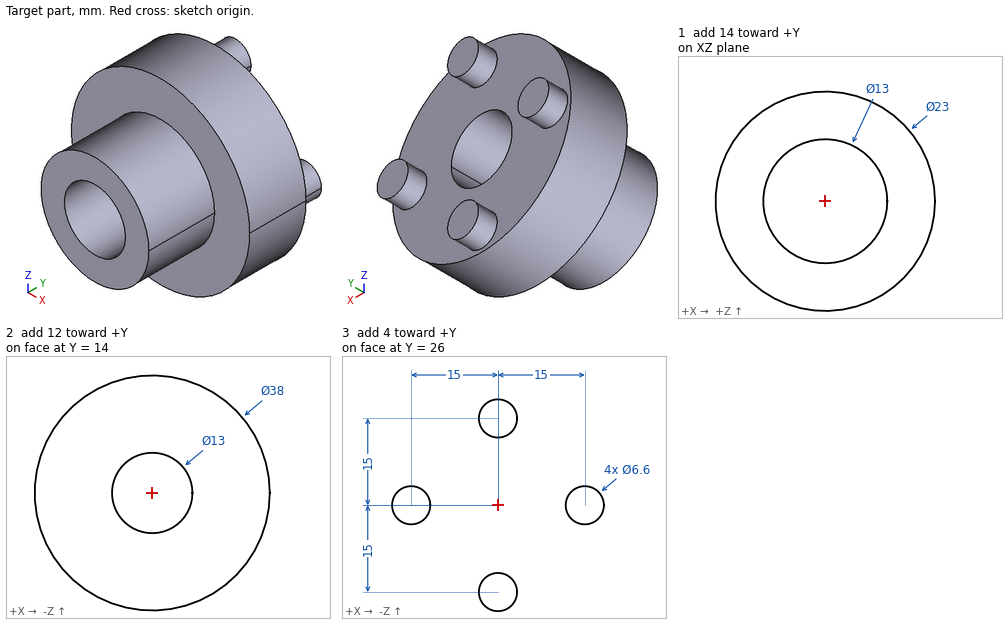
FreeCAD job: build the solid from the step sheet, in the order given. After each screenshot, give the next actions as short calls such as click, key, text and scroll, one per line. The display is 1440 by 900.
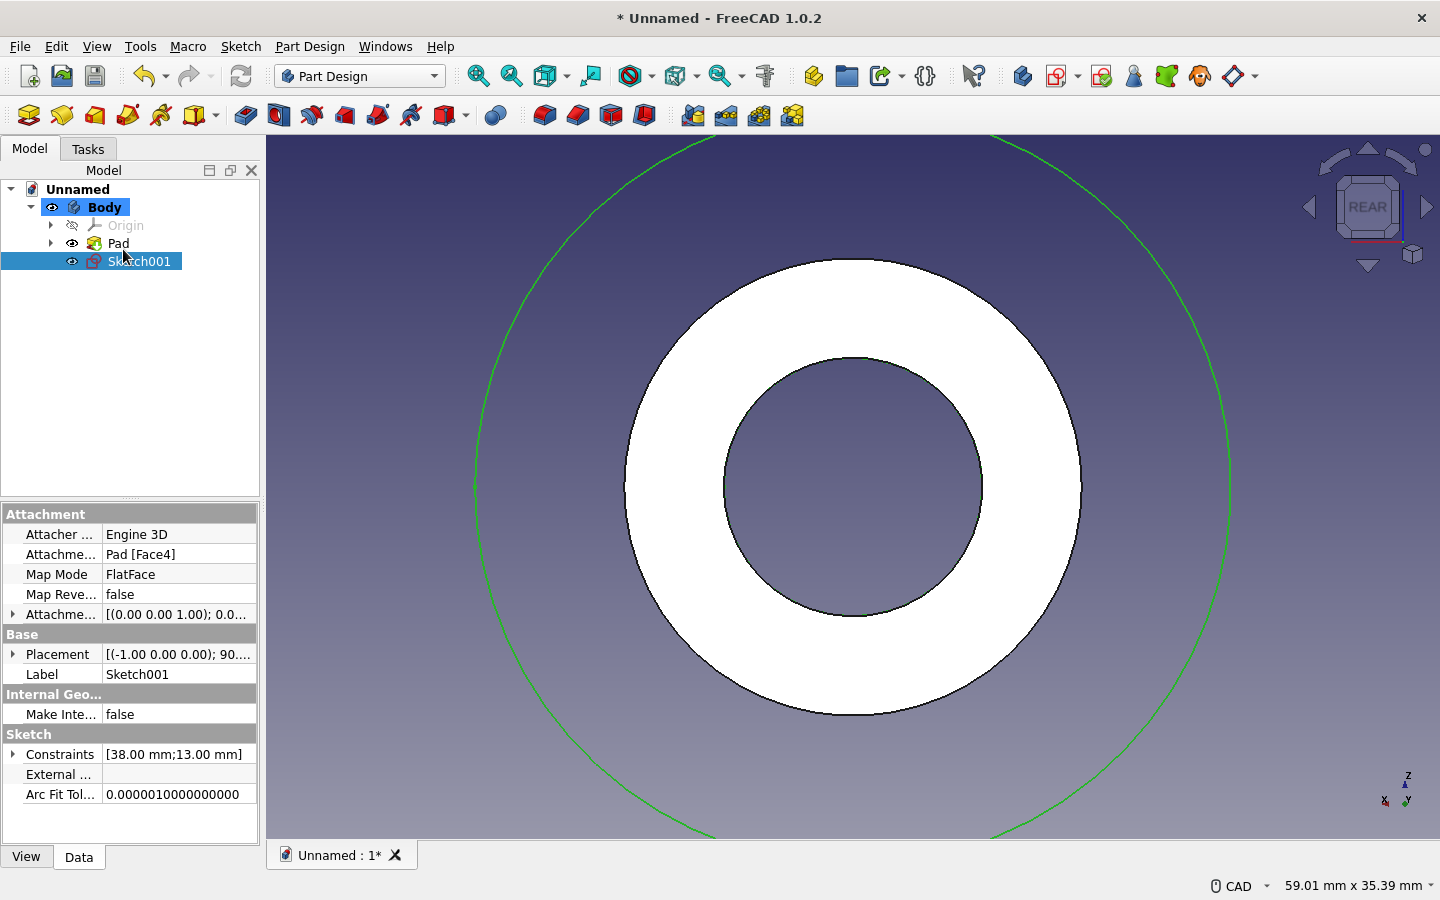
click(29, 116)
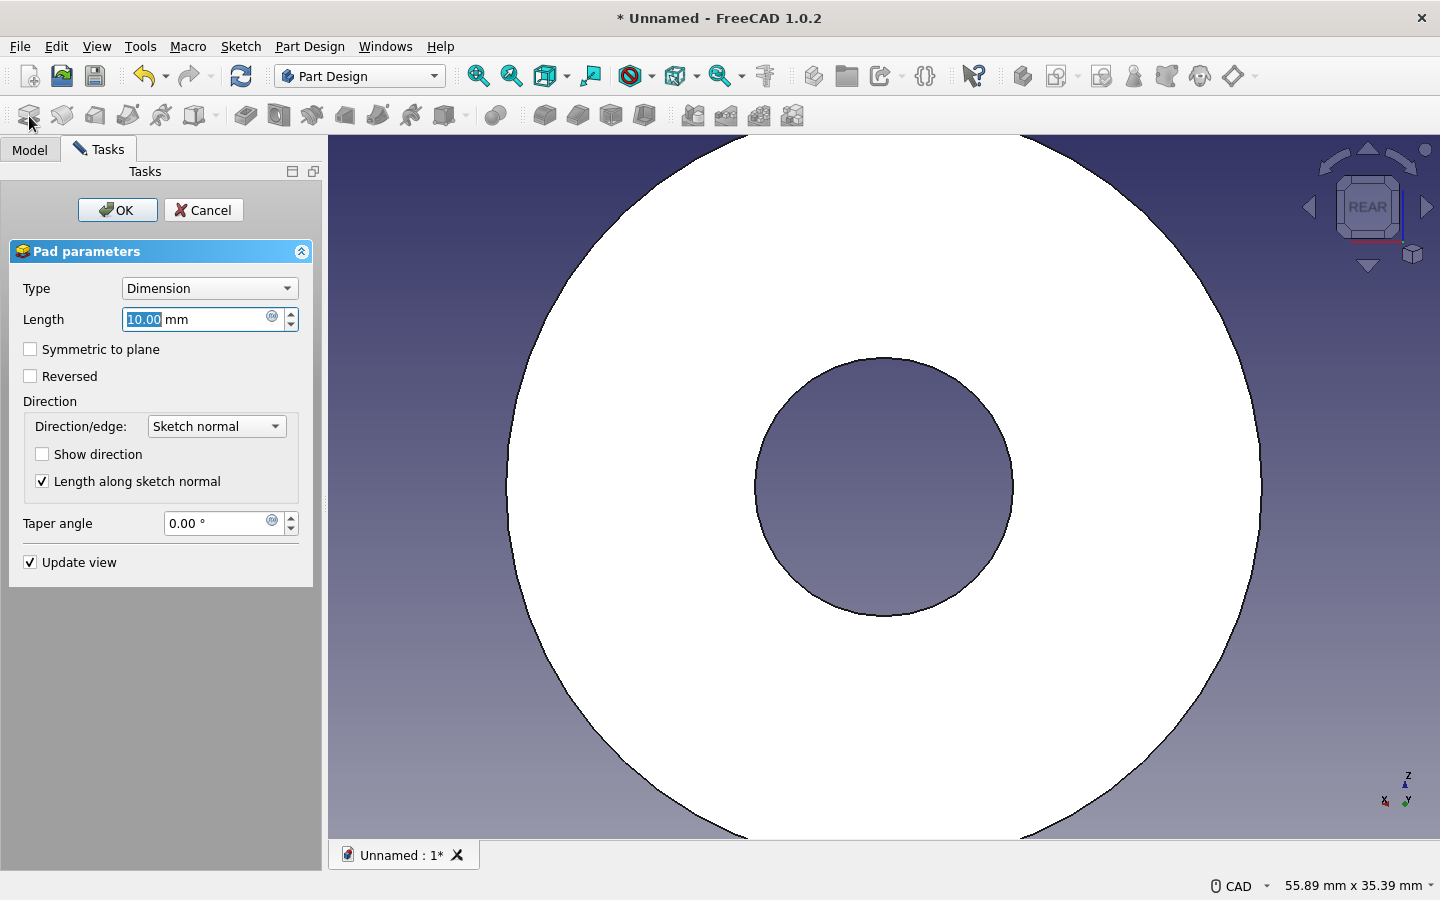
text(12)
key(Tab)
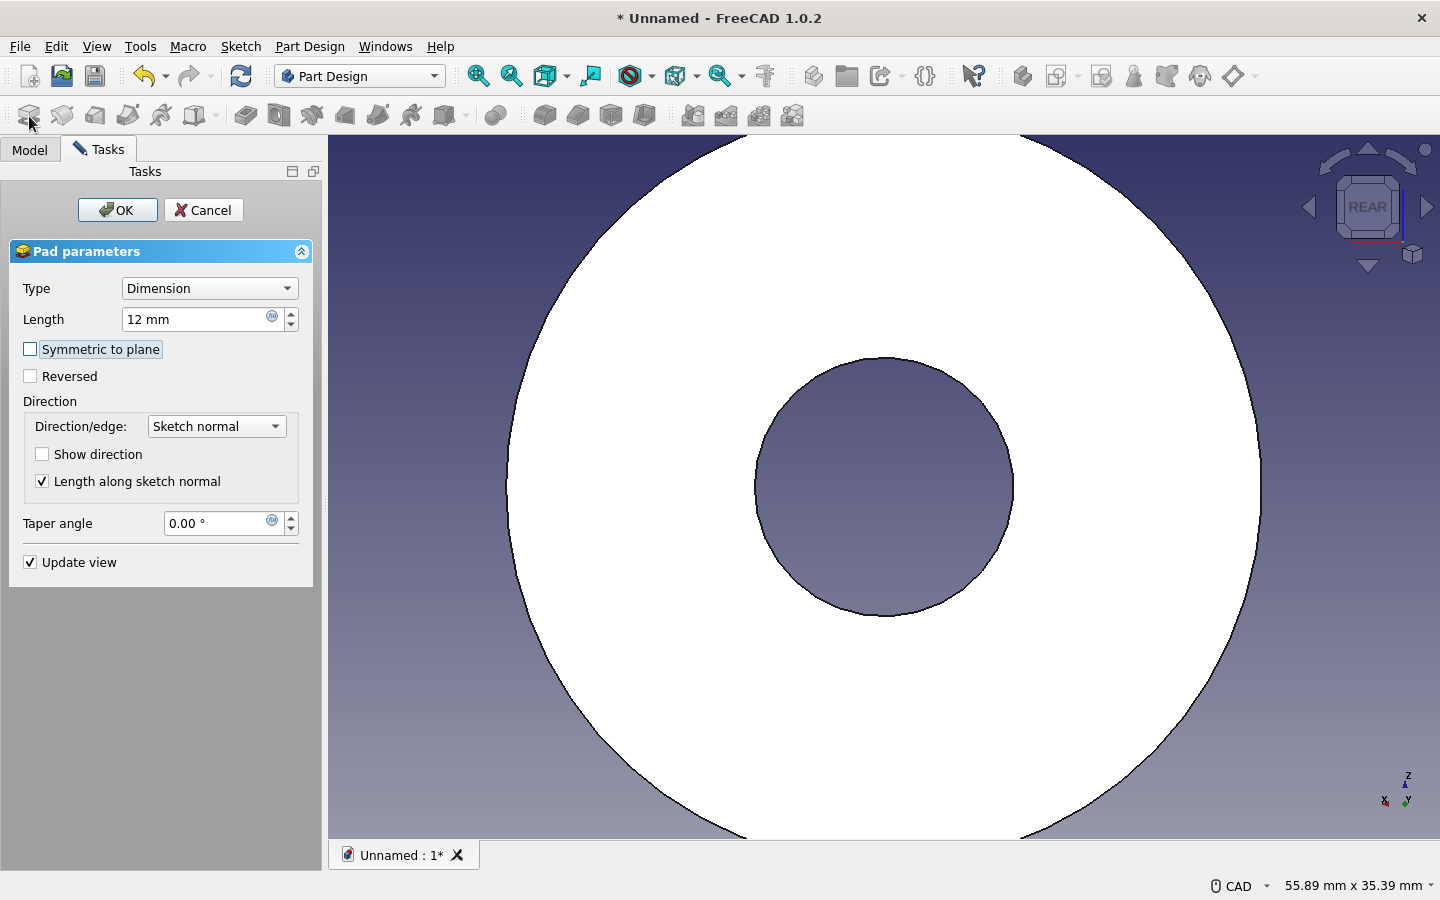
click(118, 210)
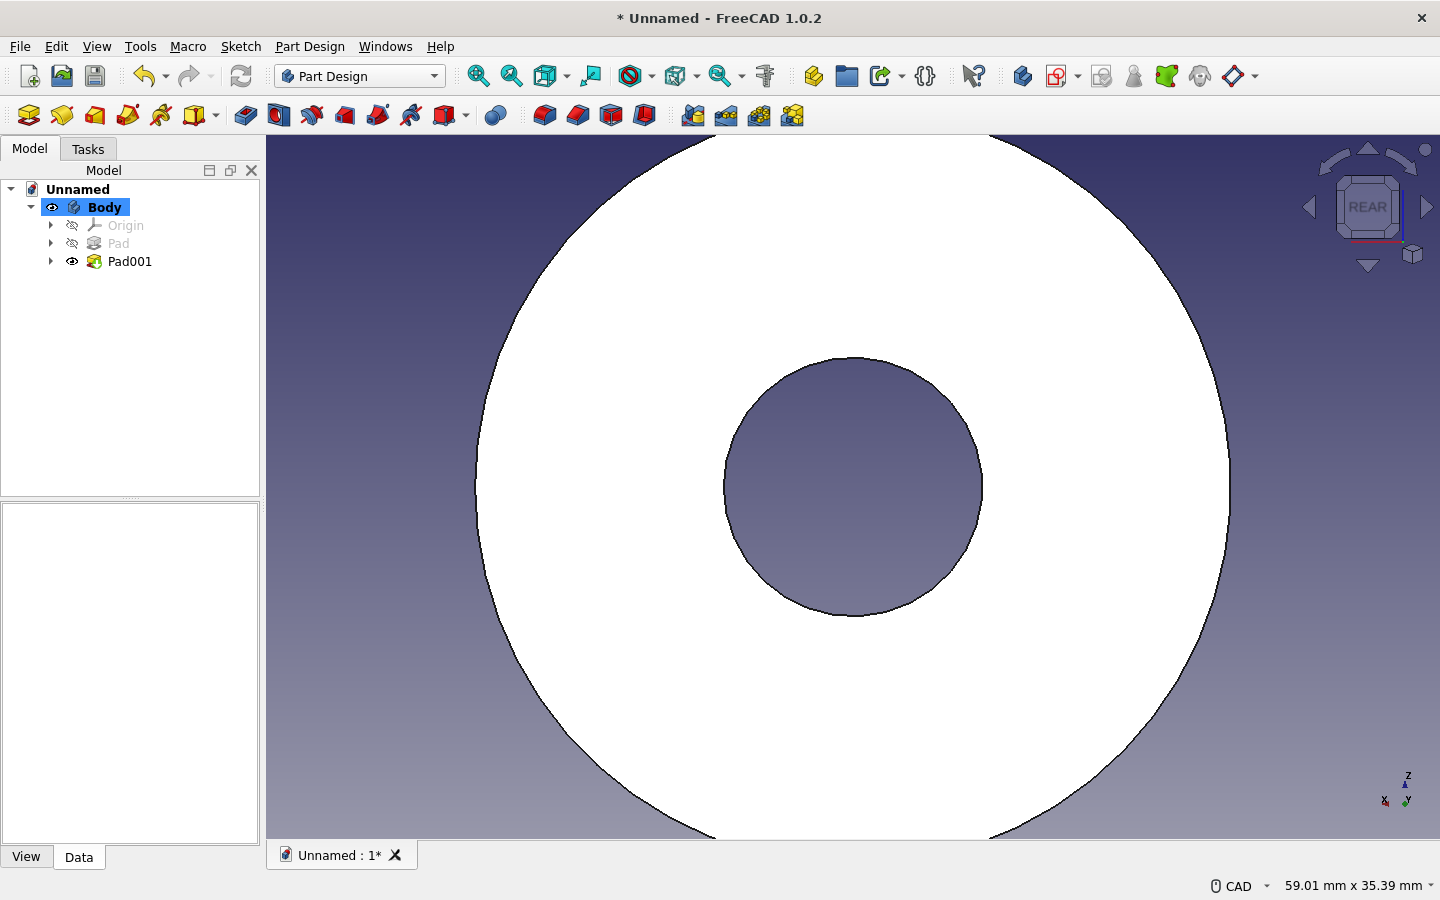
key(v)
key(f)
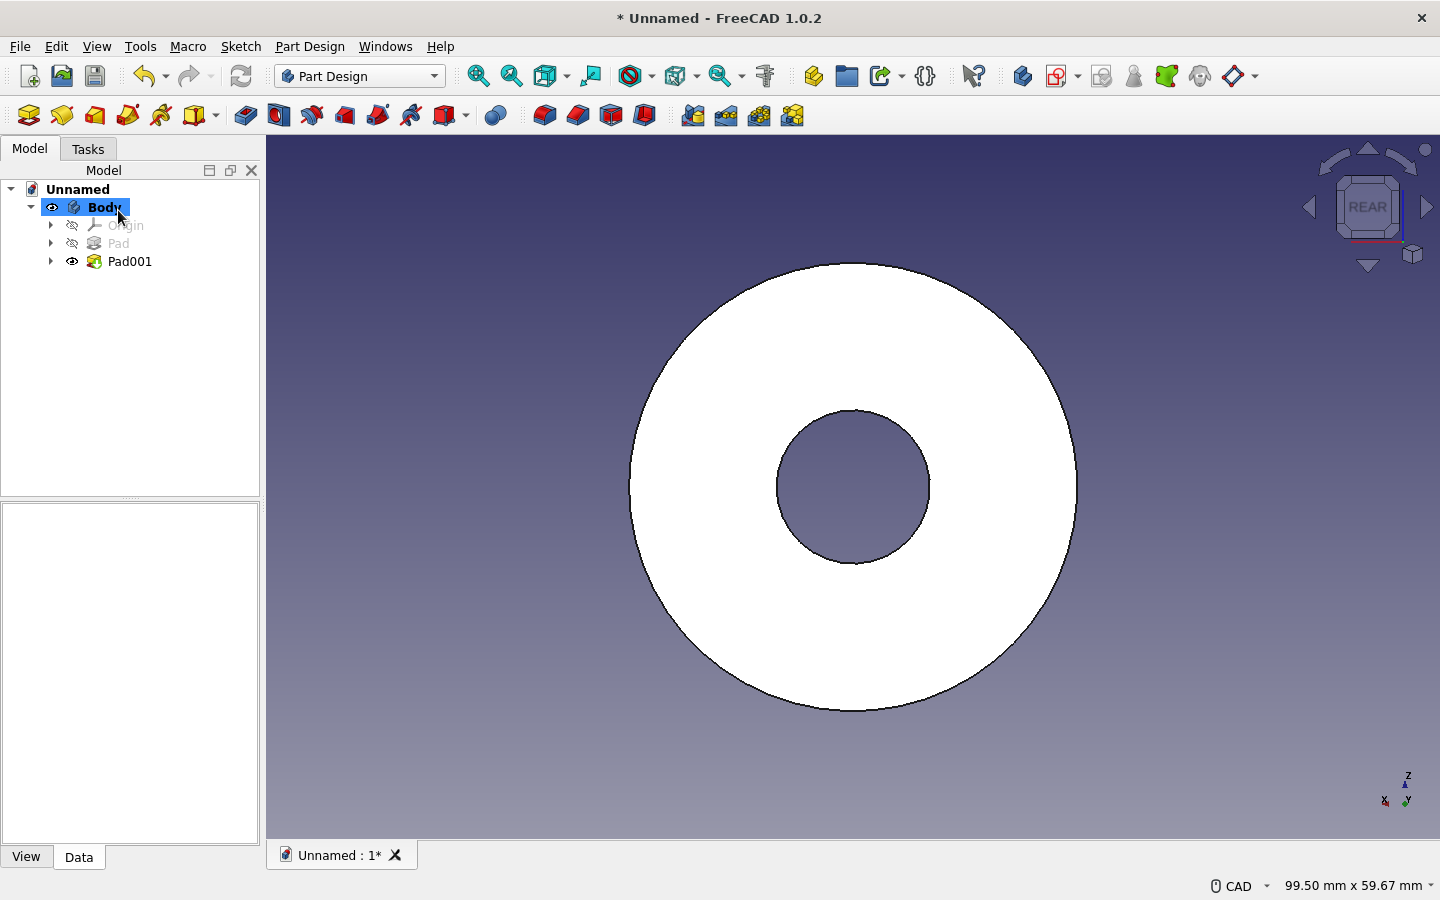
click(917, 614)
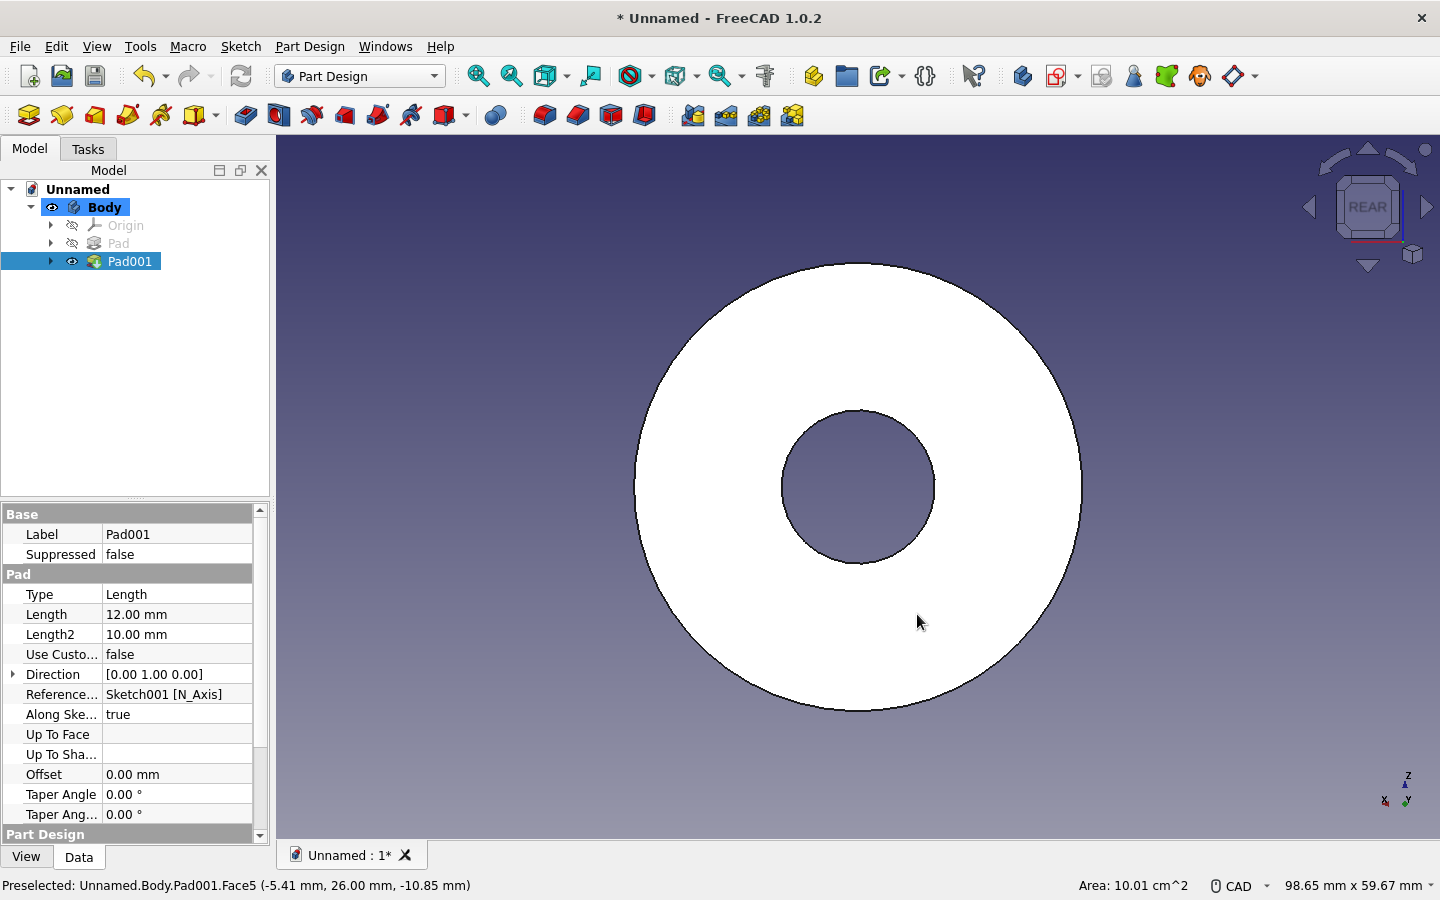
click(1056, 76)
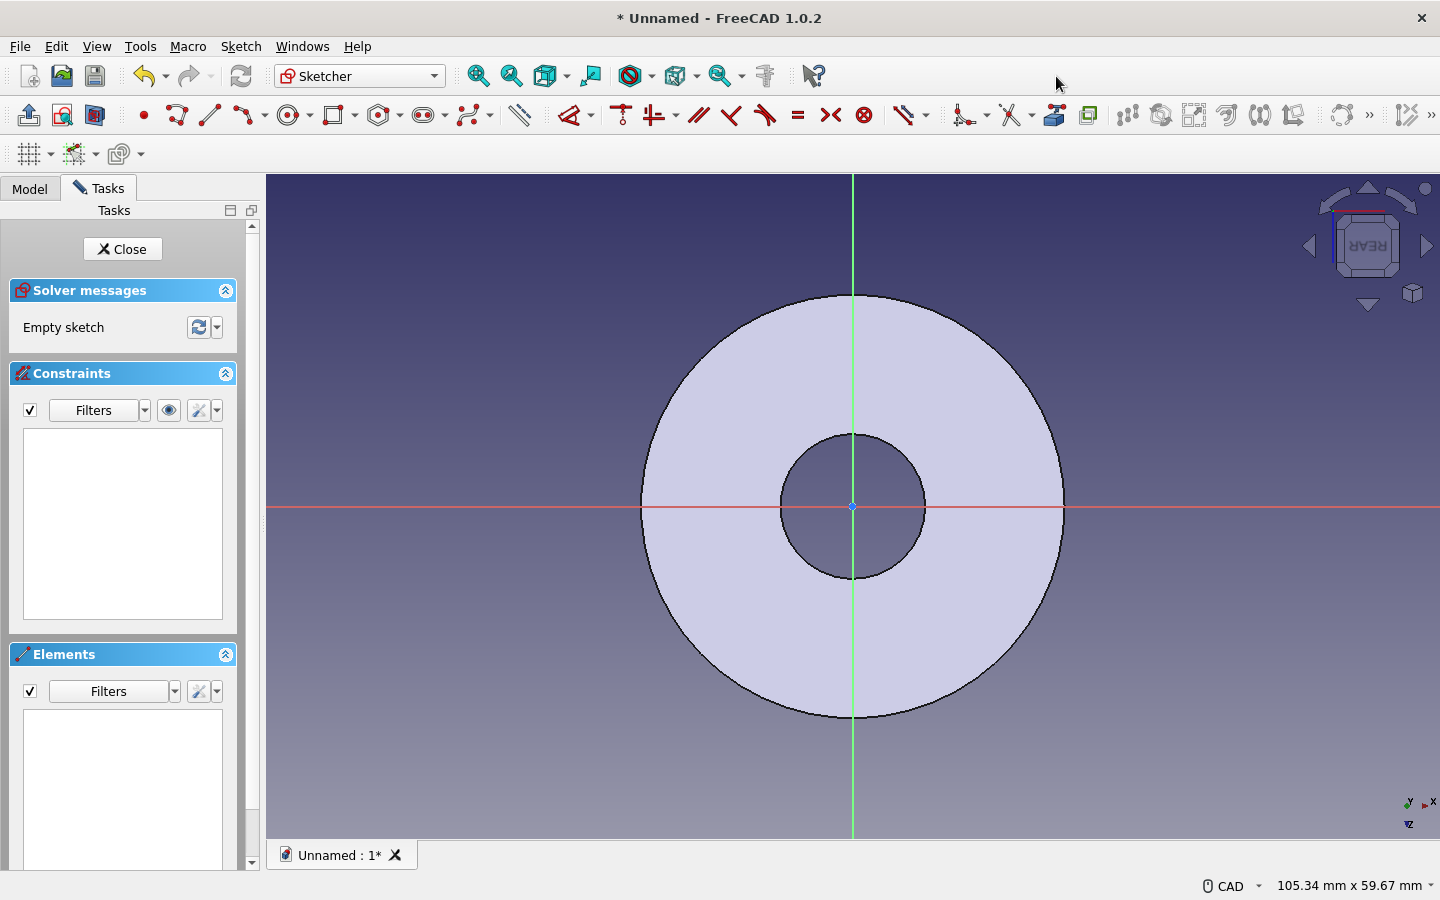
key(g)
key(c)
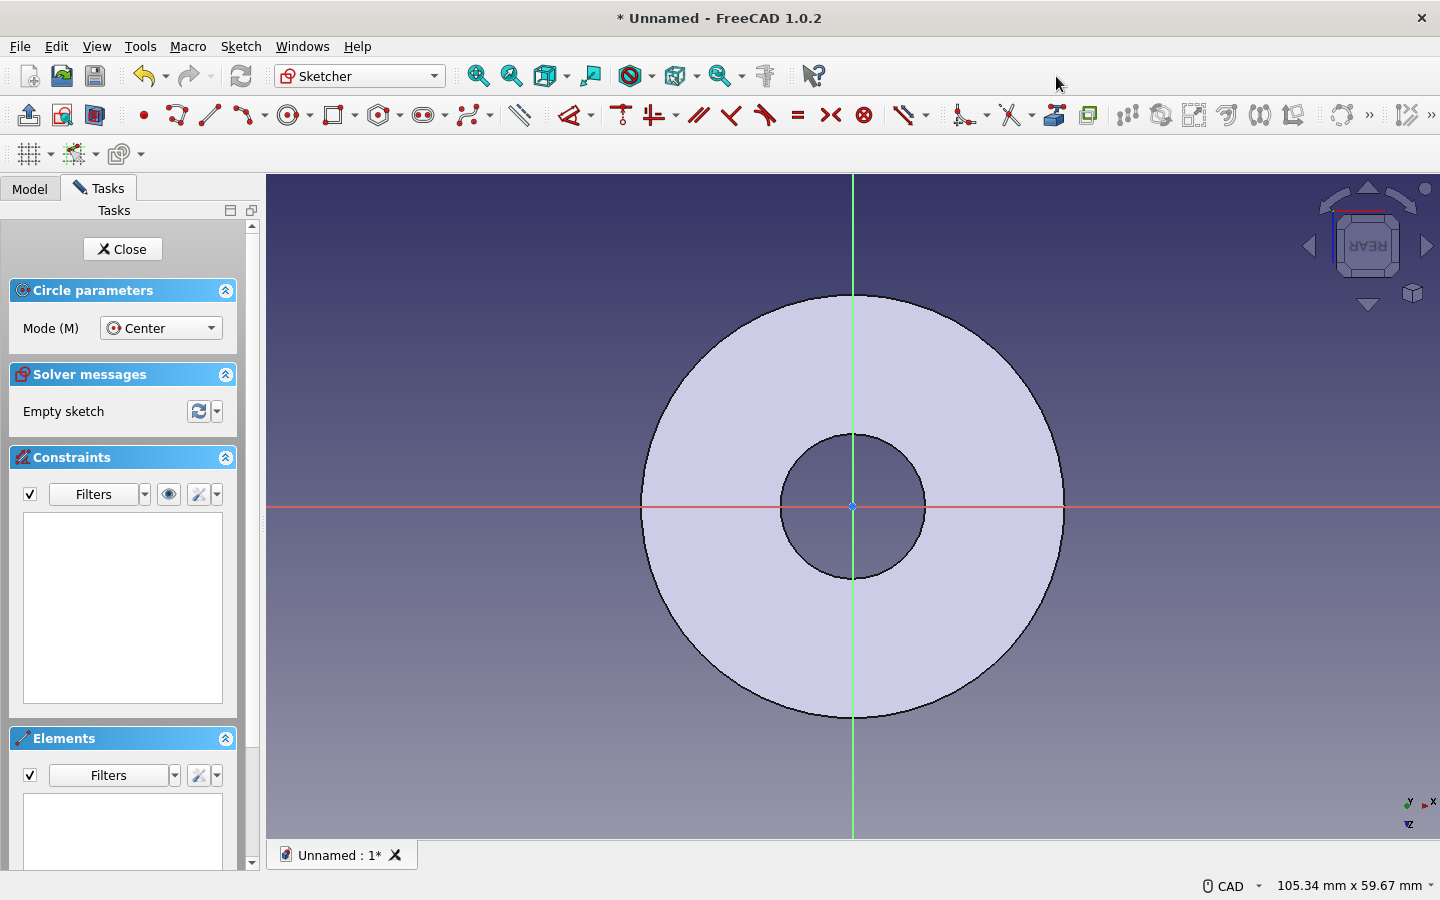
click(1020, 506)
click(1046, 480)